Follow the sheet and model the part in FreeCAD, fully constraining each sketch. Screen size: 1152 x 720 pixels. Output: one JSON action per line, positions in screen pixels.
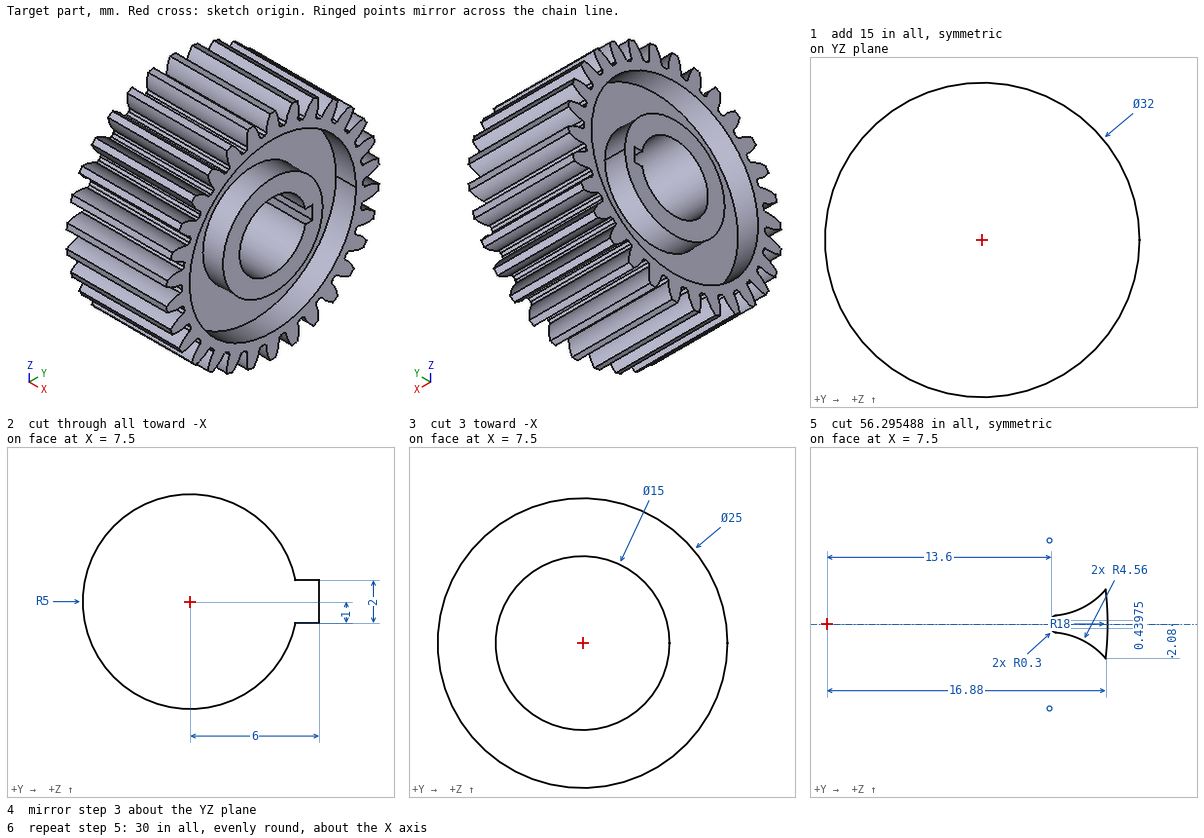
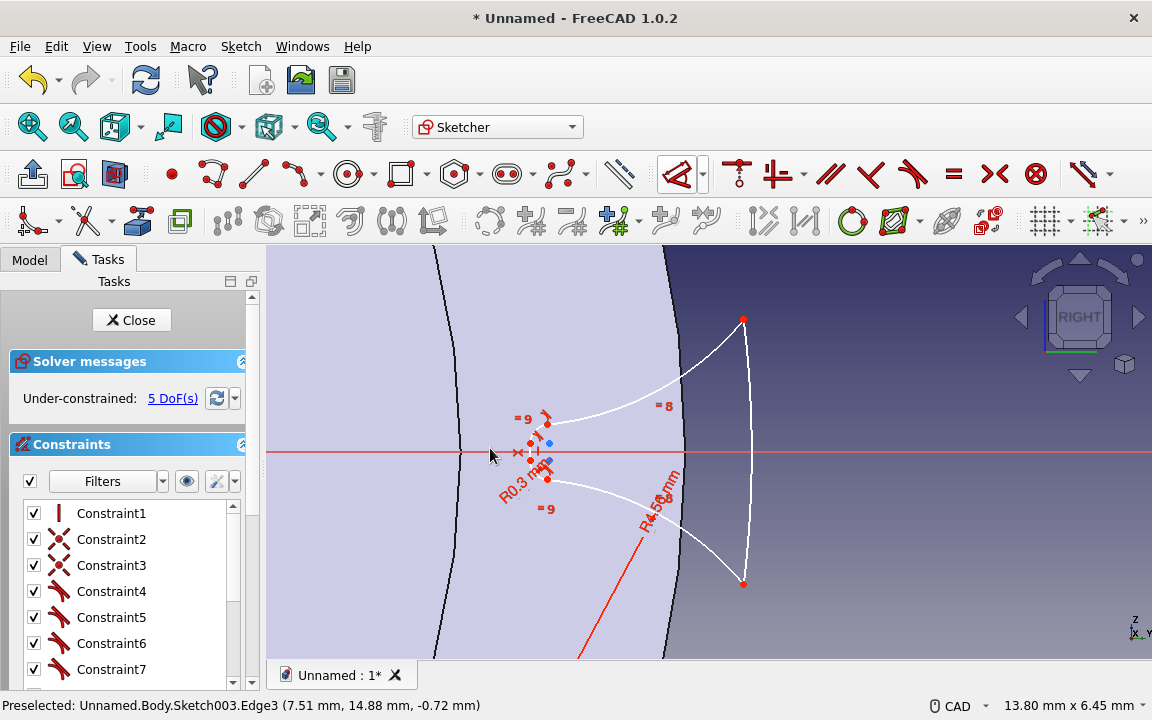
{"action": "left_click", "coordinate": [750, 505]}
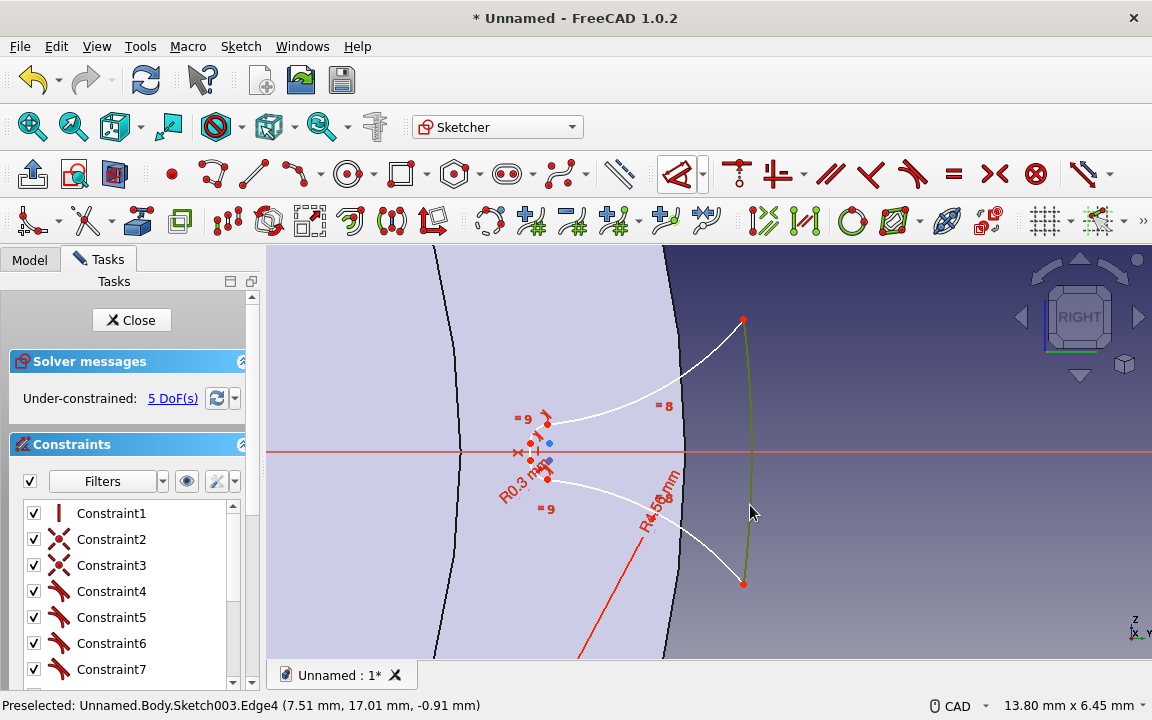
{"action": "key", "text": "k r"}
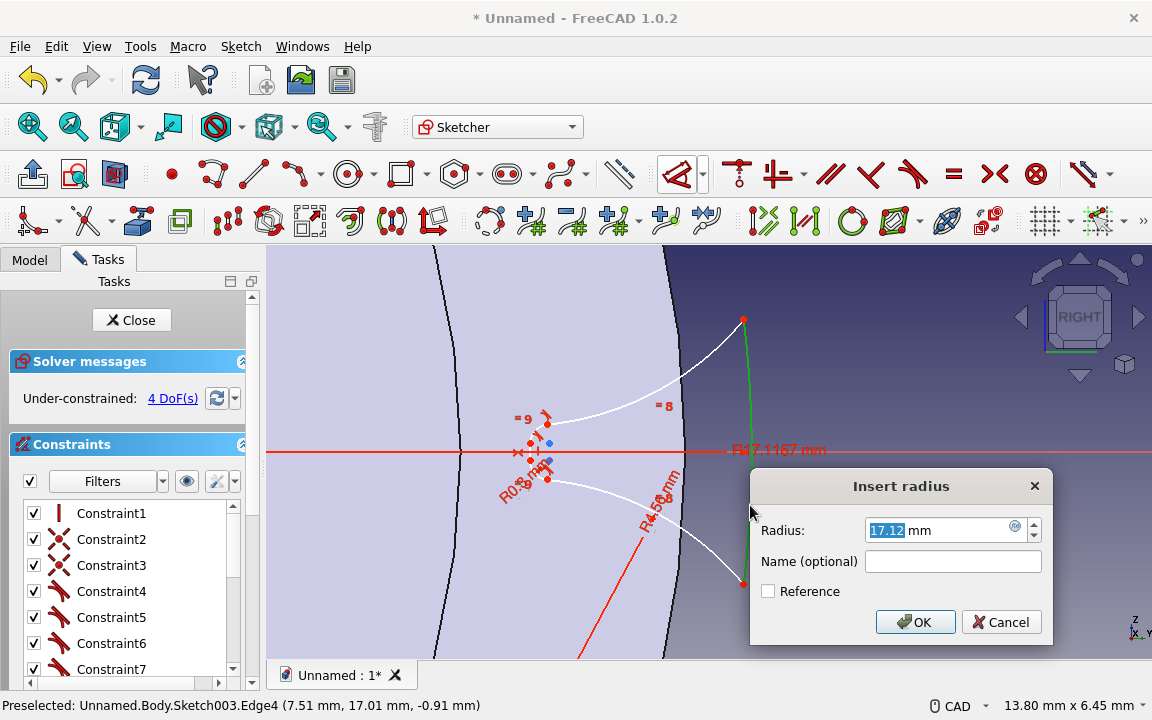
{"action": "type", "text": "18"}
{"action": "key", "text": "Return"}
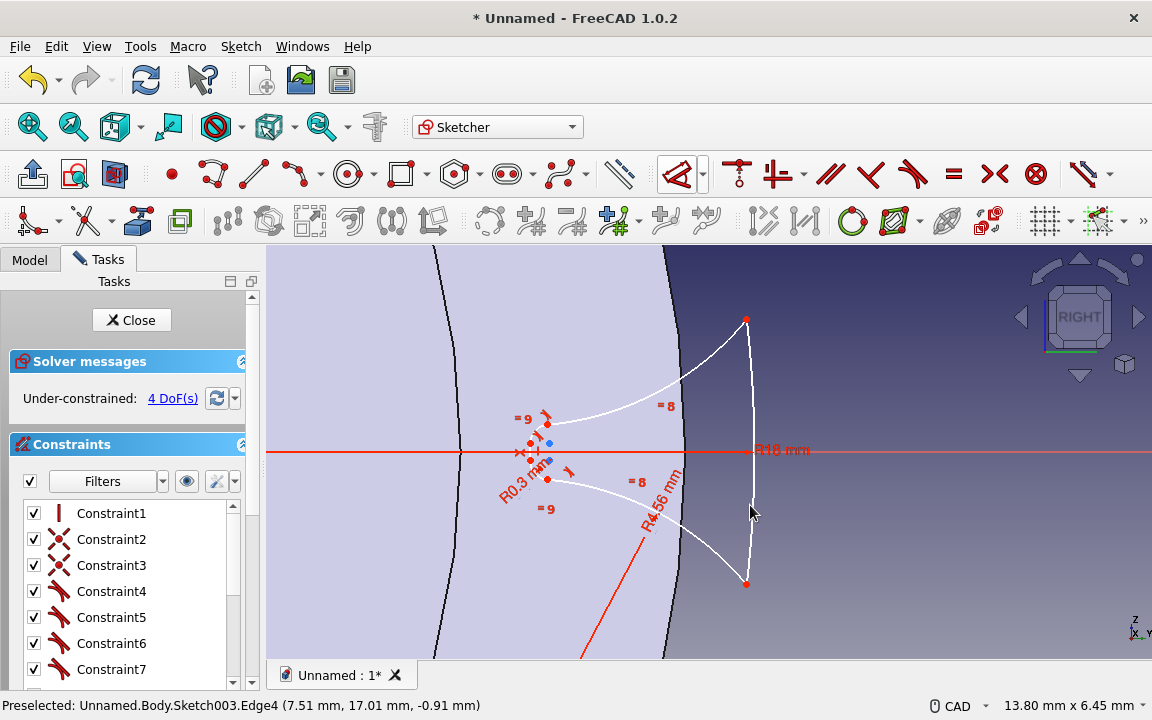
{"action": "left_click", "coordinate": [530, 444]}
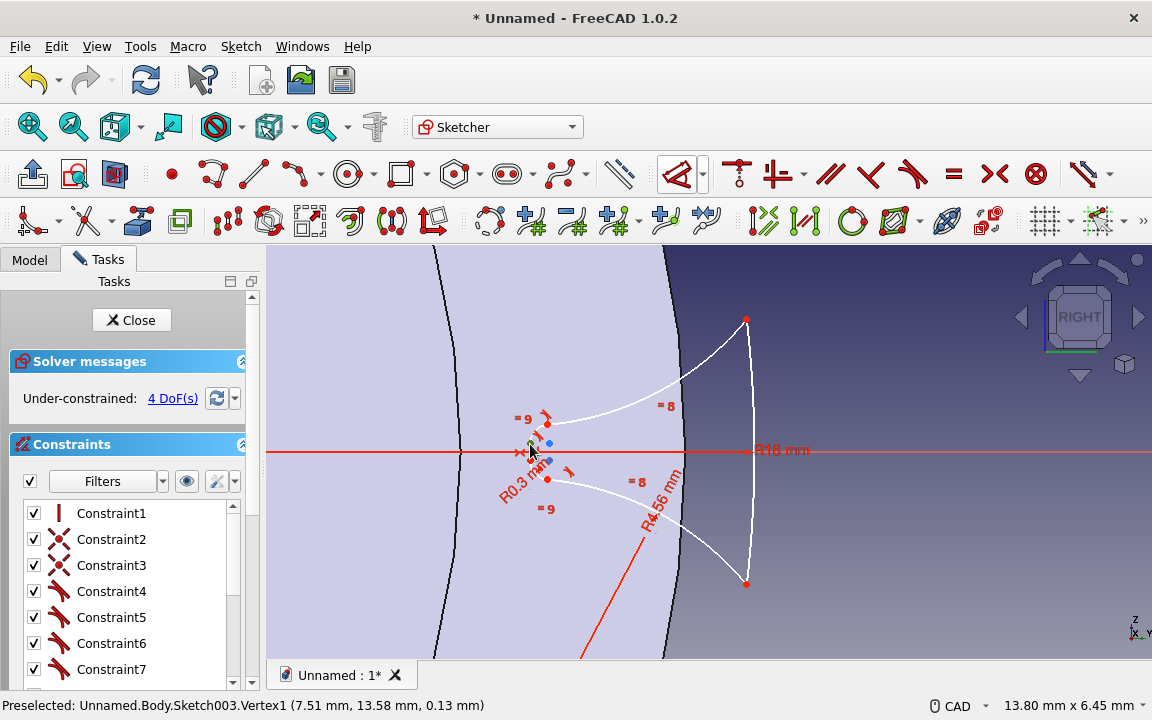
{"action": "key", "text": "l"}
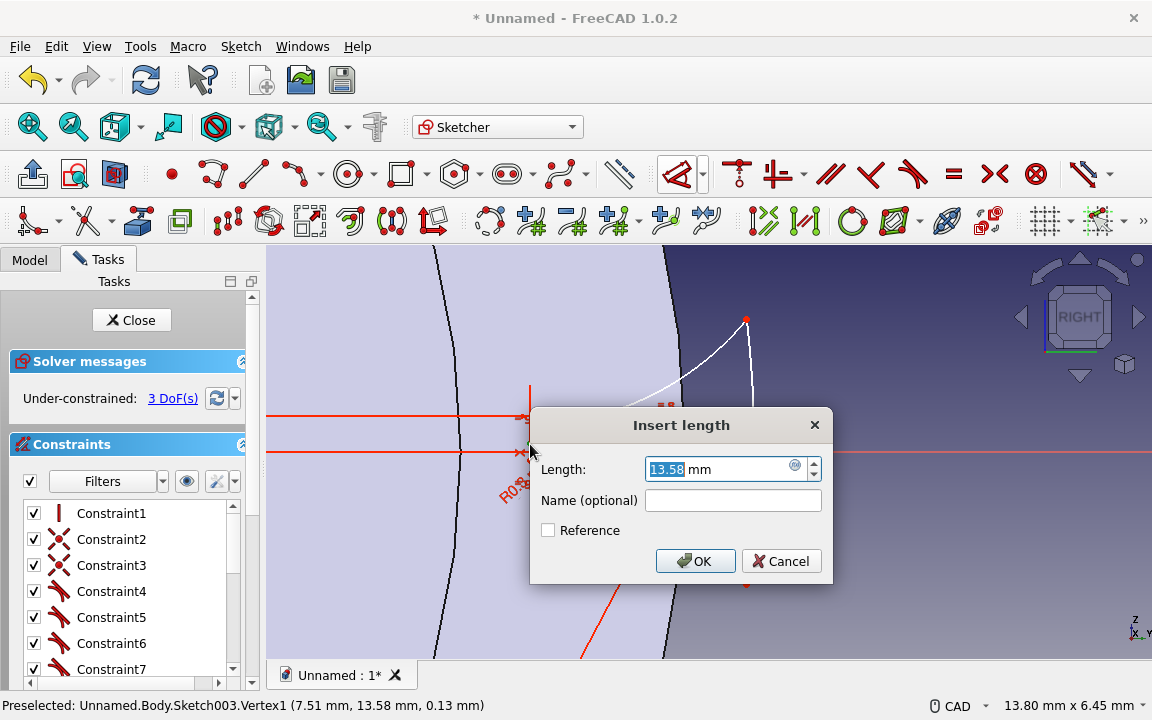
{"action": "type", "text": "13.6"}
{"action": "key", "text": "Return"}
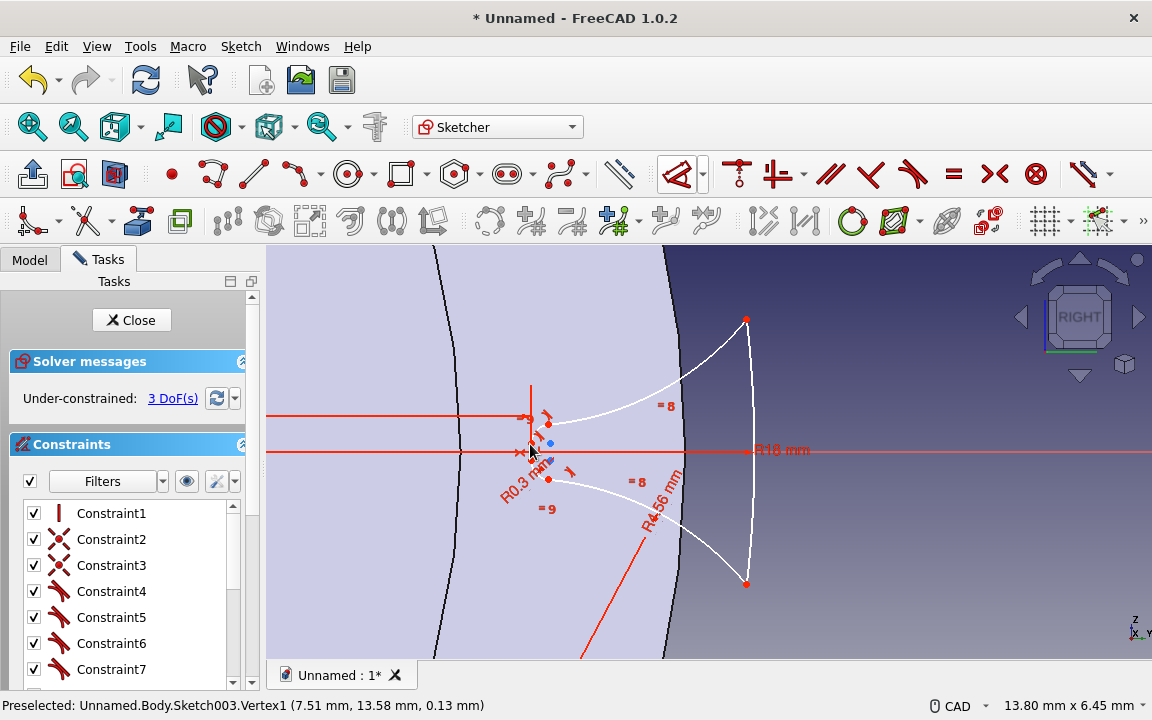
{"action": "left_click", "coordinate": [747, 585]}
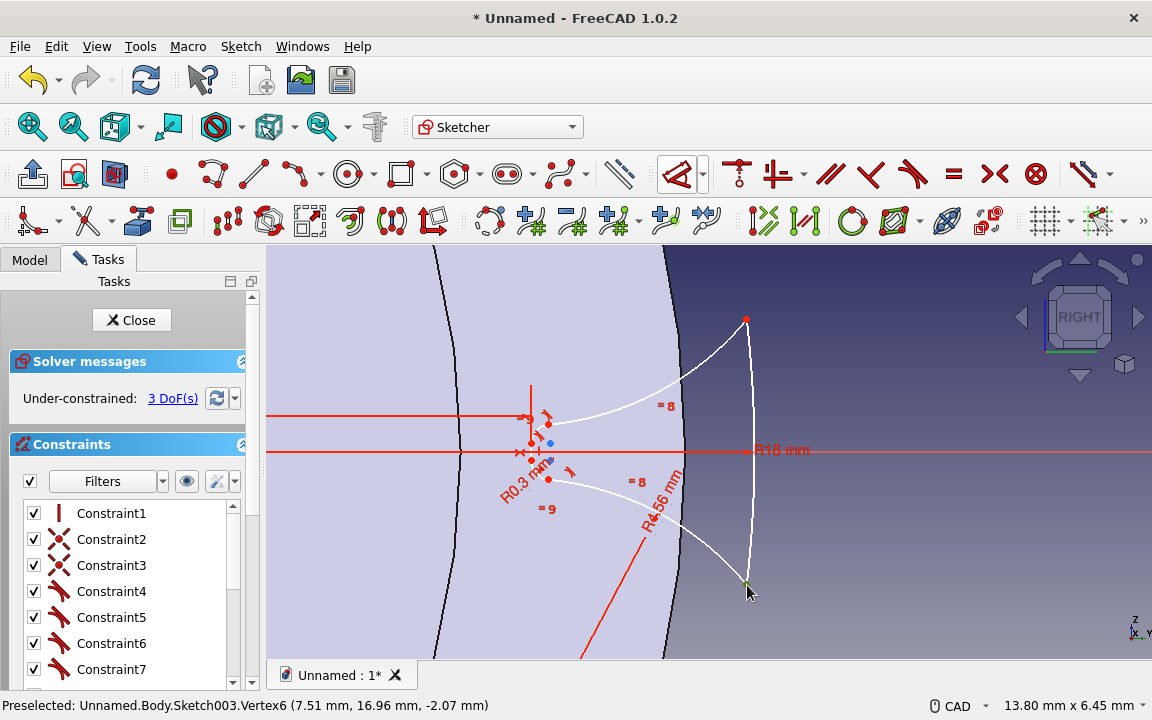
{"action": "key", "text": "i"}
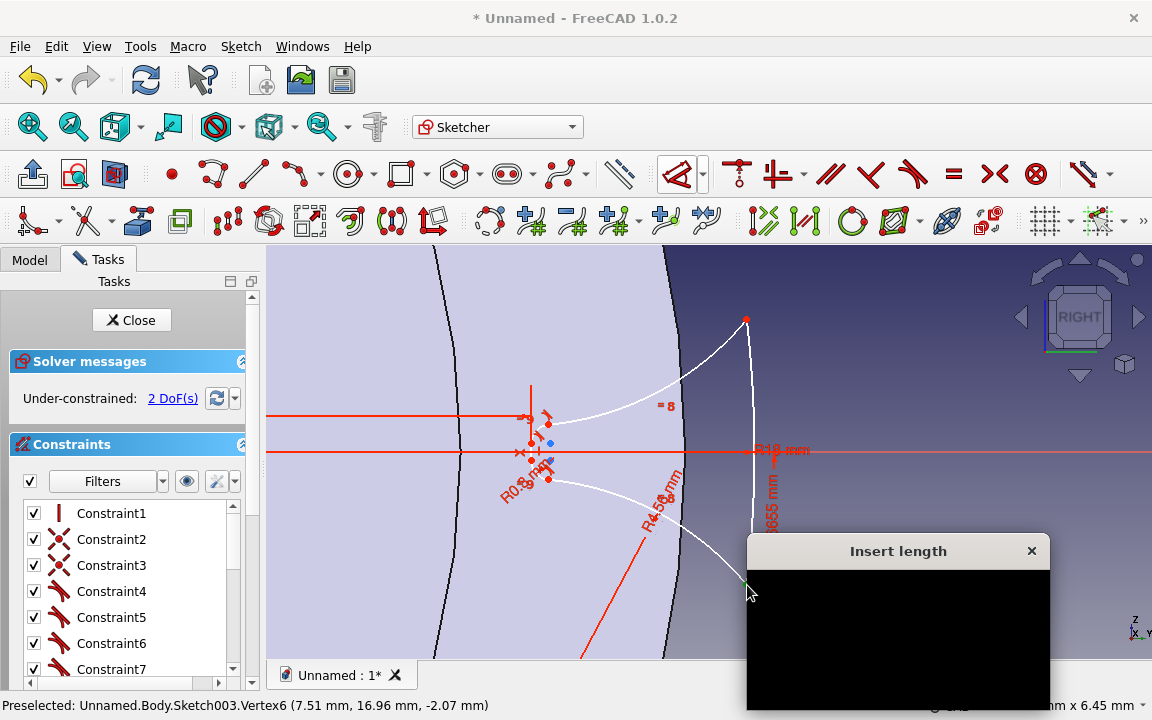
{"action": "type", "text": "-2.08"}
{"action": "key", "text": "Return"}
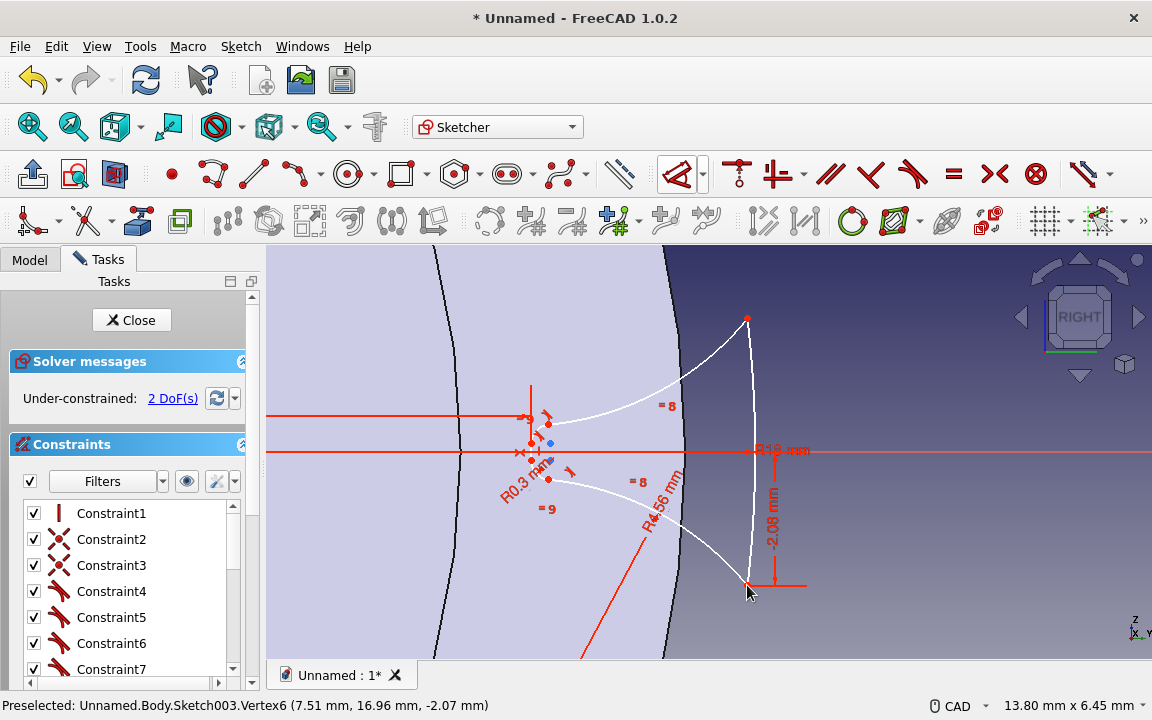
{"action": "left_click", "coordinate": [747, 586]}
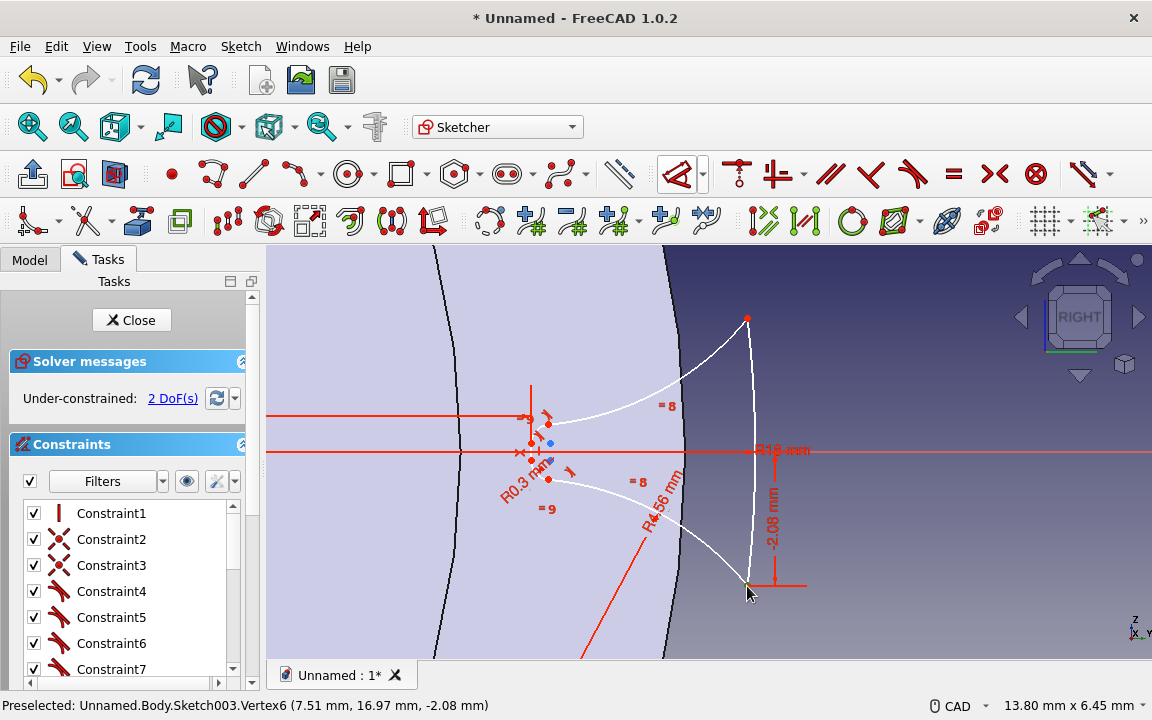
{"action": "key", "text": "l"}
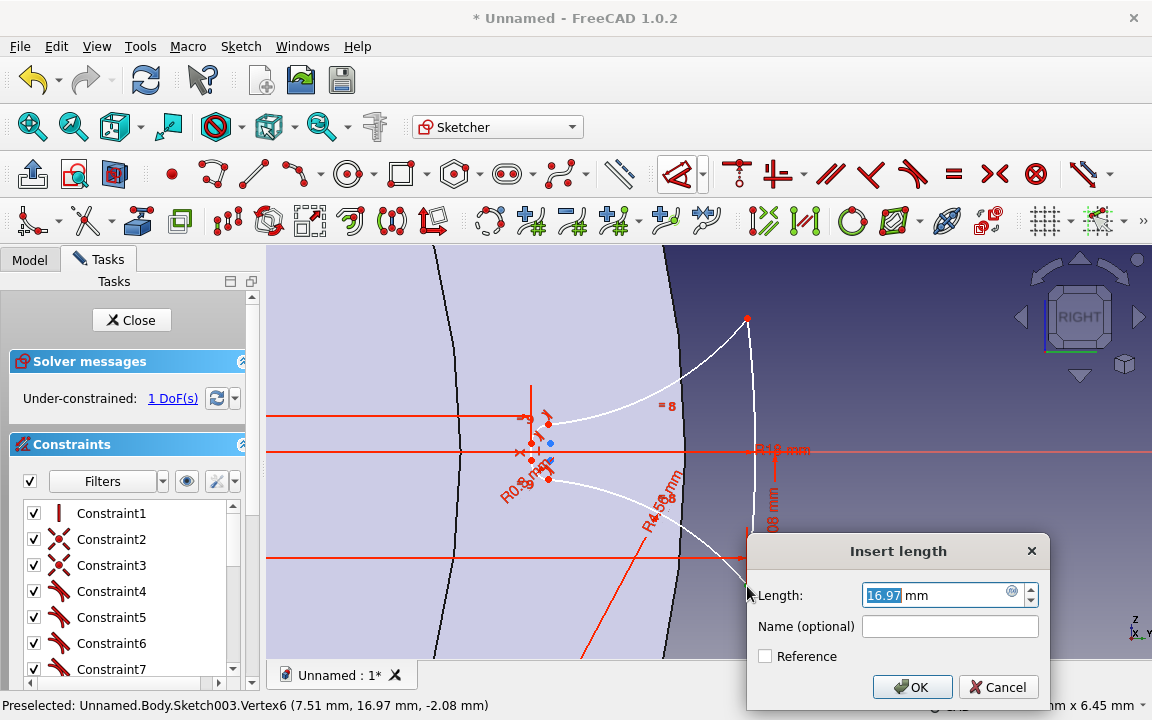
{"action": "type", "text": "16.88"}
{"action": "key", "text": "Return"}